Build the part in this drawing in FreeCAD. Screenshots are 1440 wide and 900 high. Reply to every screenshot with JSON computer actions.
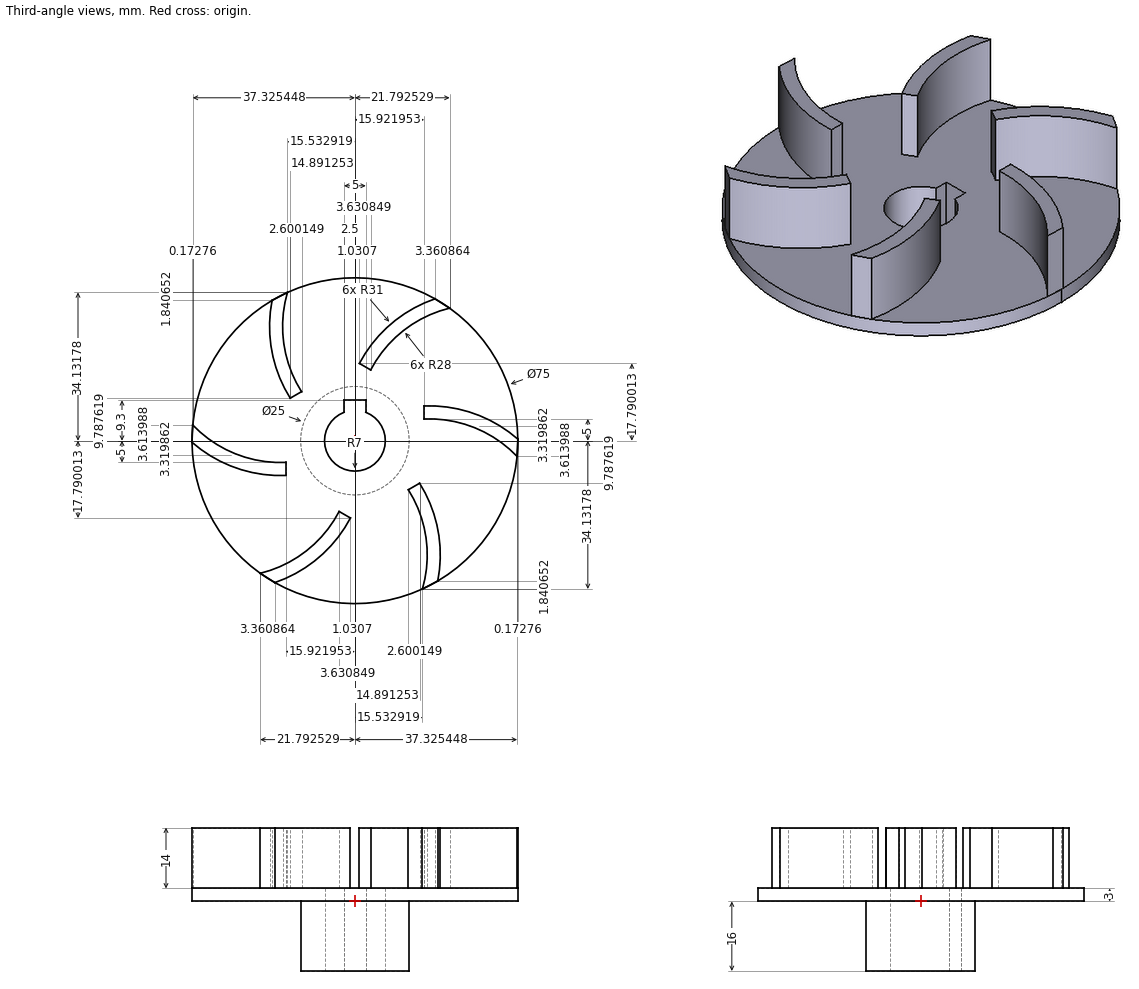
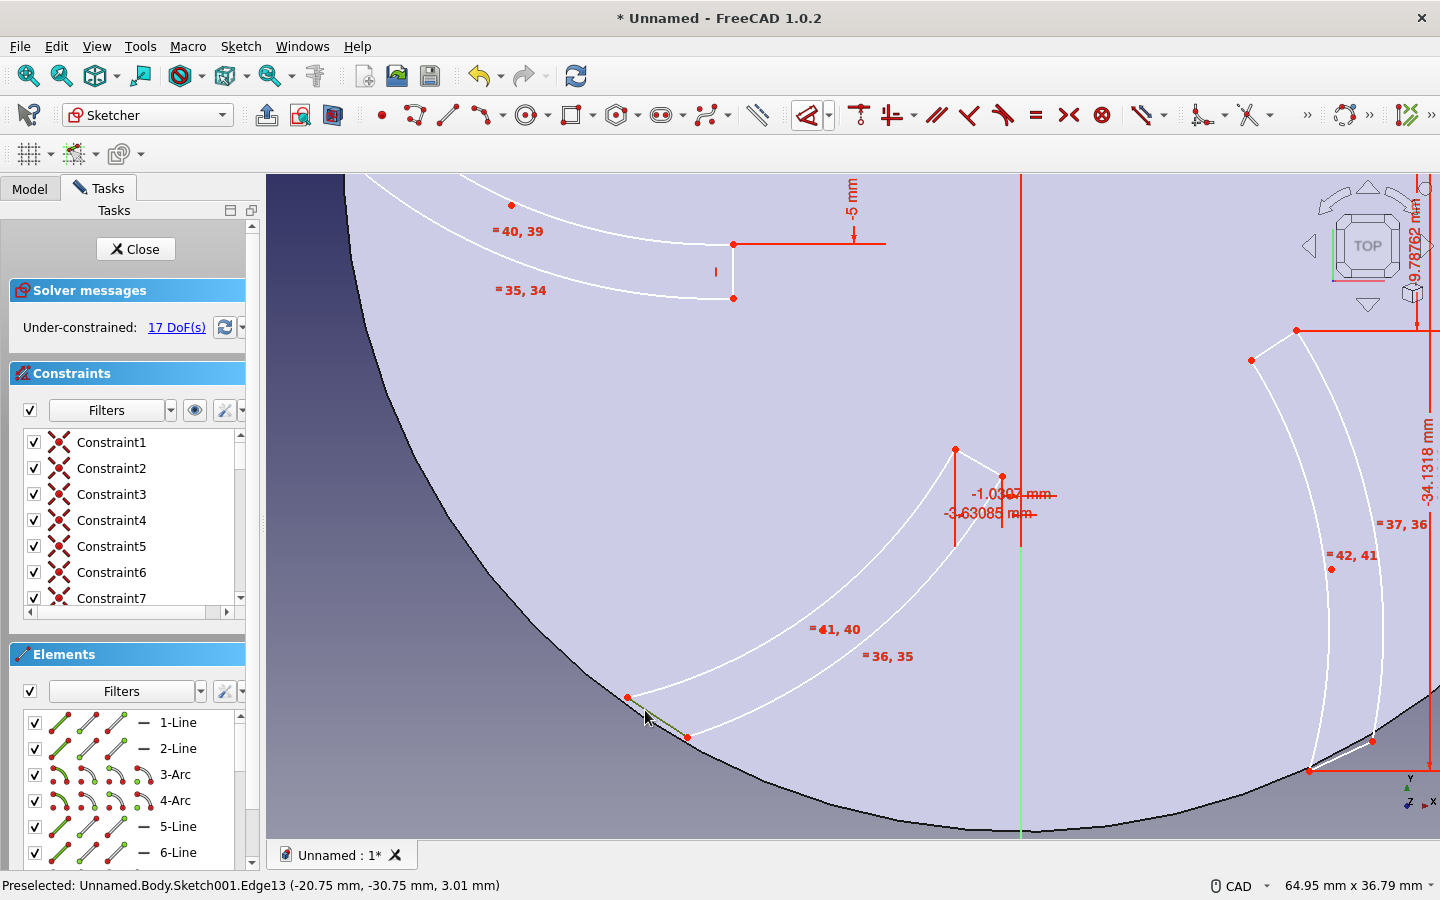
{"action": "key", "text": "l"}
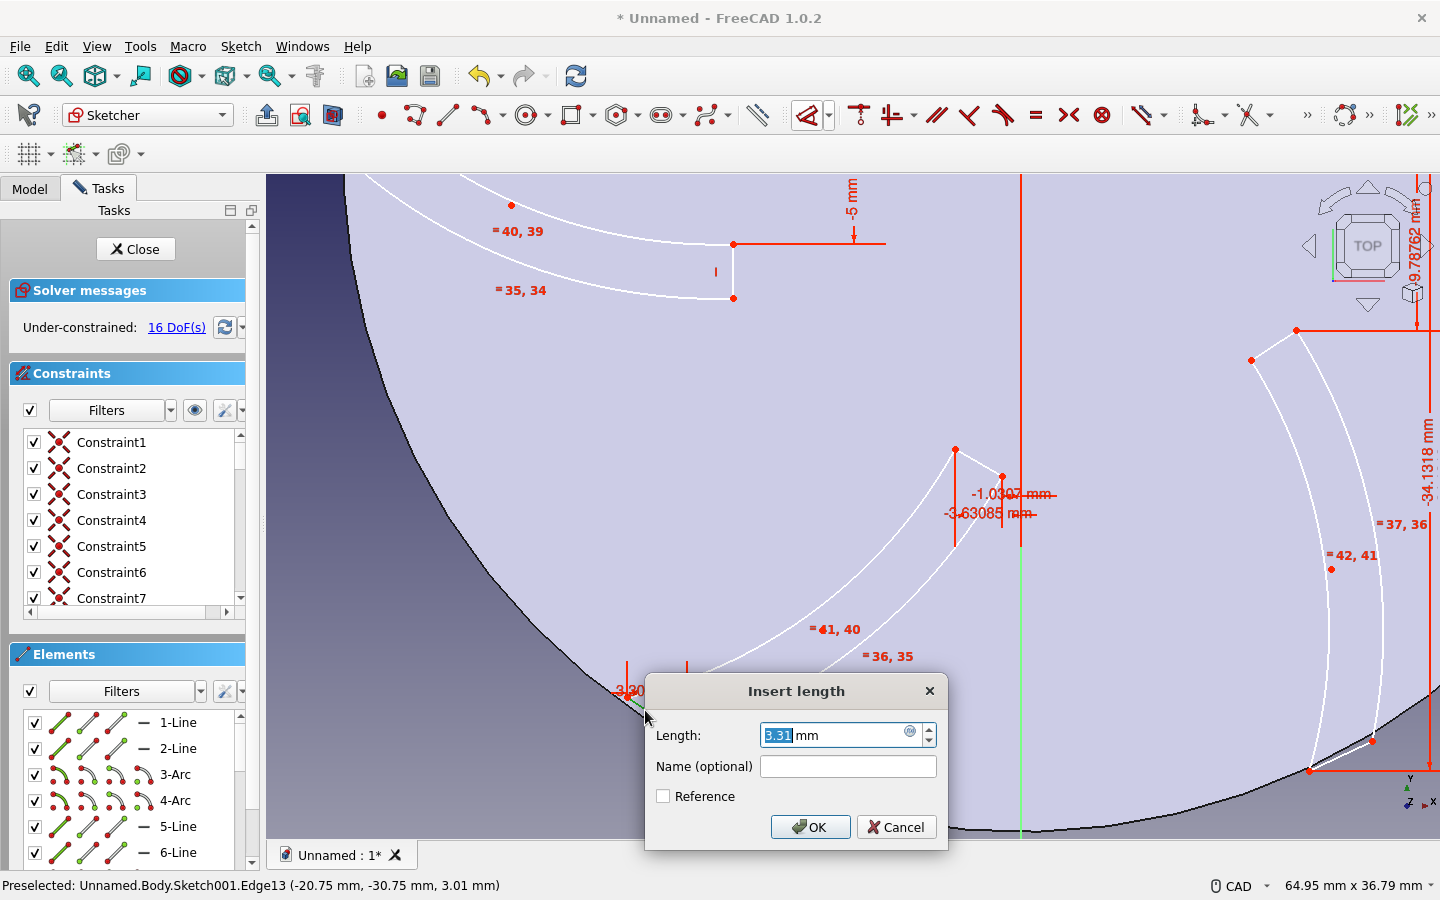
{"action": "type", "text": "3.360864"}
{"action": "key", "text": "Return"}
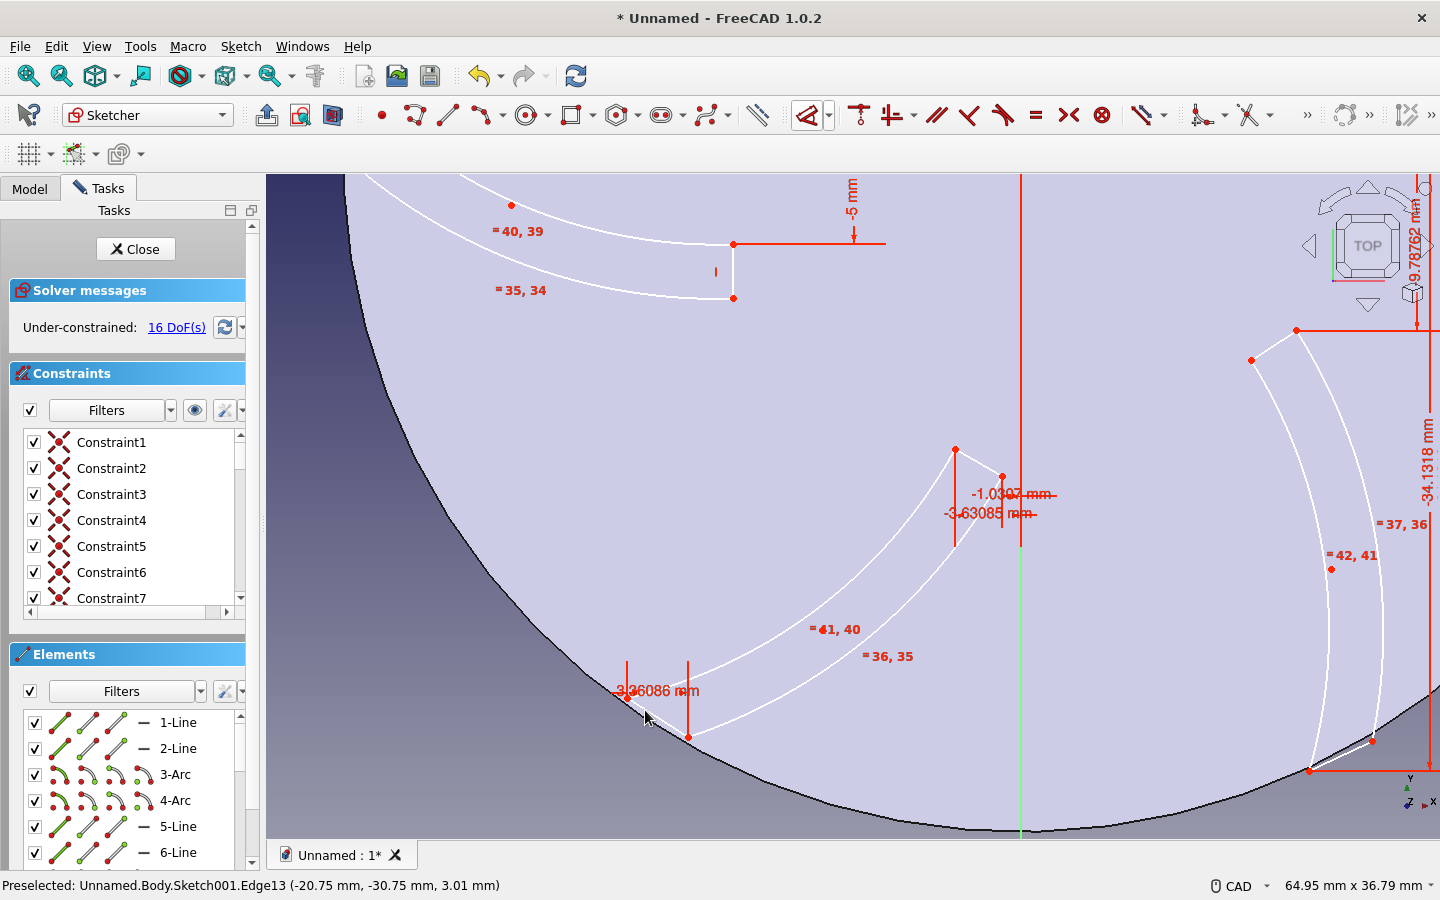
{"action": "scroll", "coordinate": [647, 712], "scroll_direction": "down", "scroll_amount": 5}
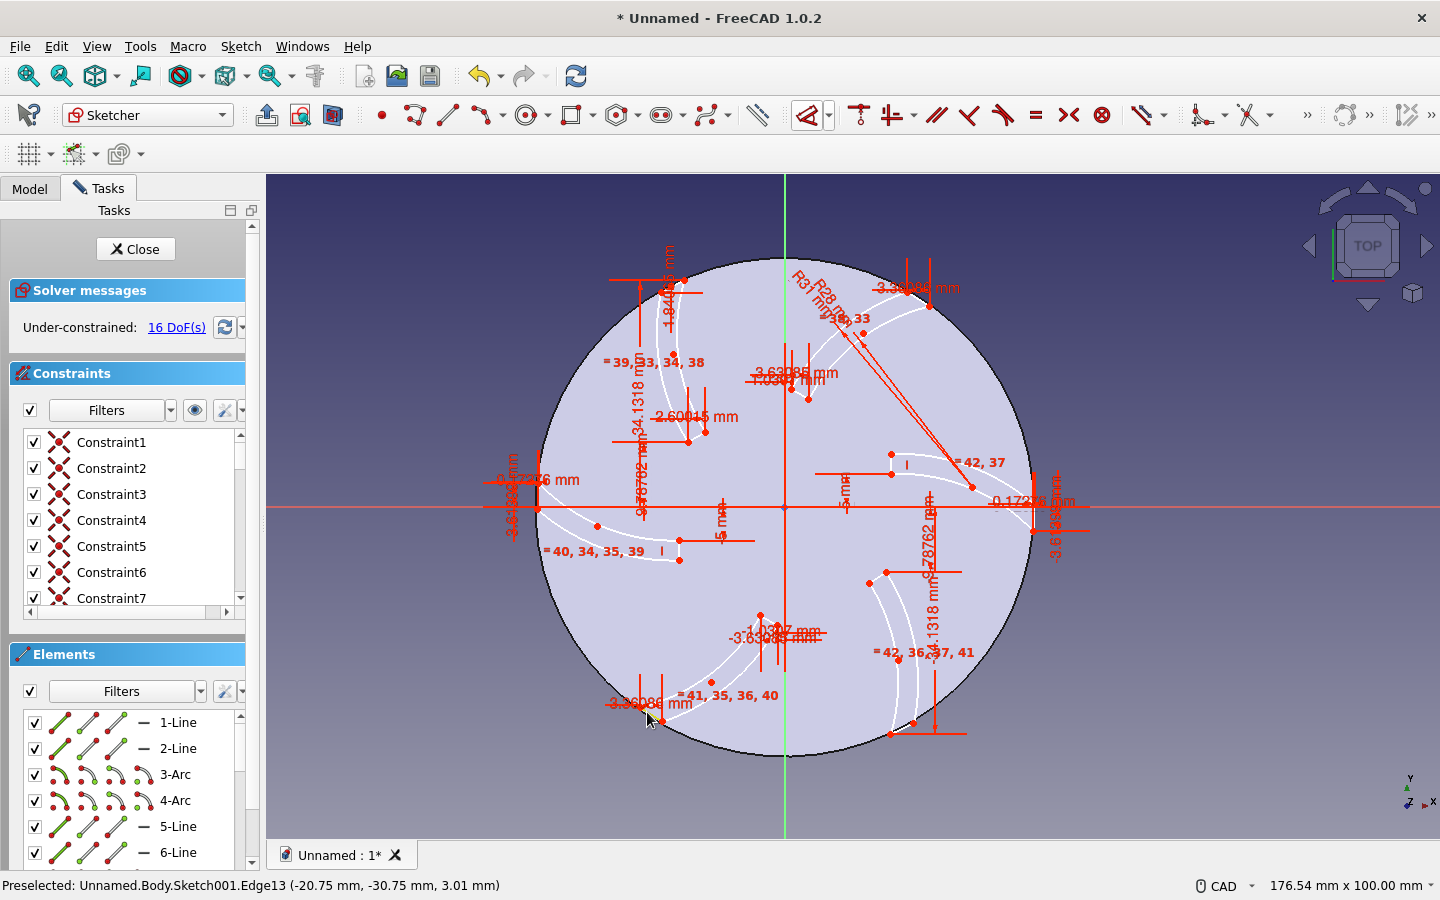
{"action": "scroll", "coordinate": [898, 731], "scroll_direction": "up", "scroll_amount": 6}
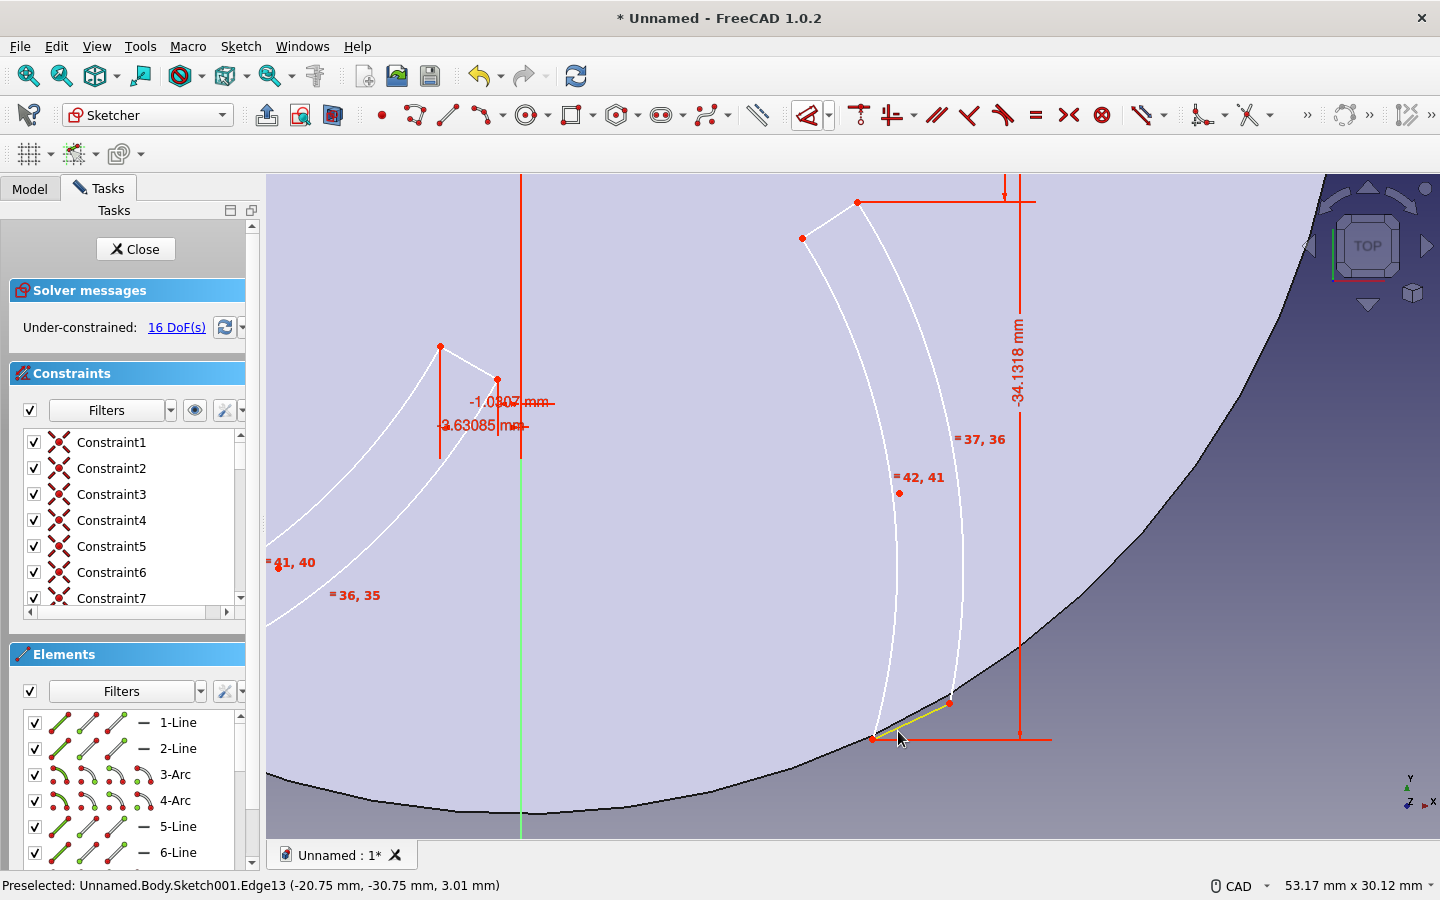
{"action": "left_click", "coordinate": [896, 729]}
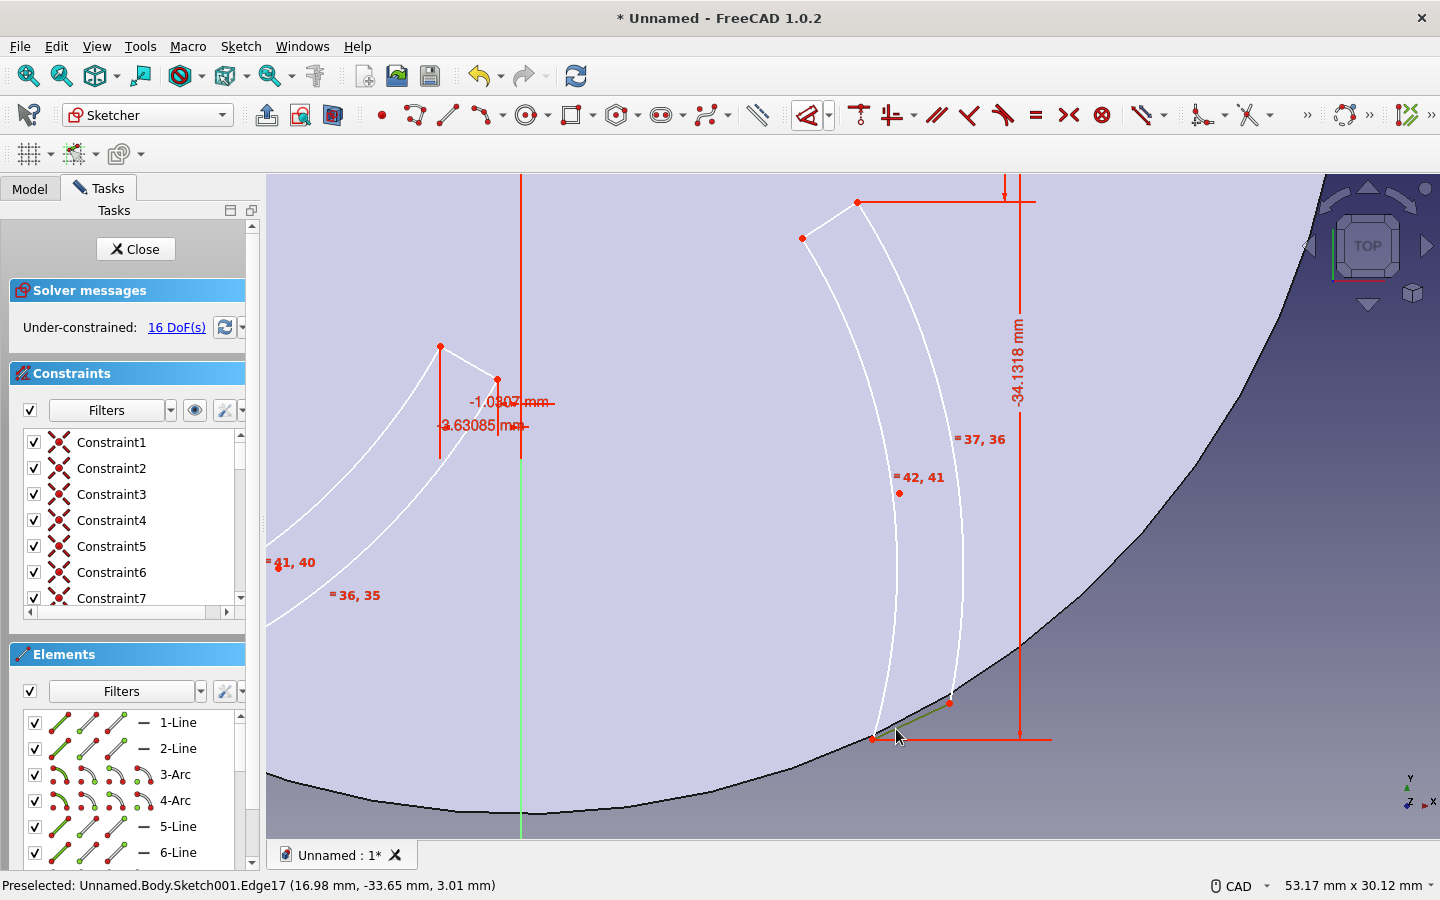
{"action": "key", "text": "i"}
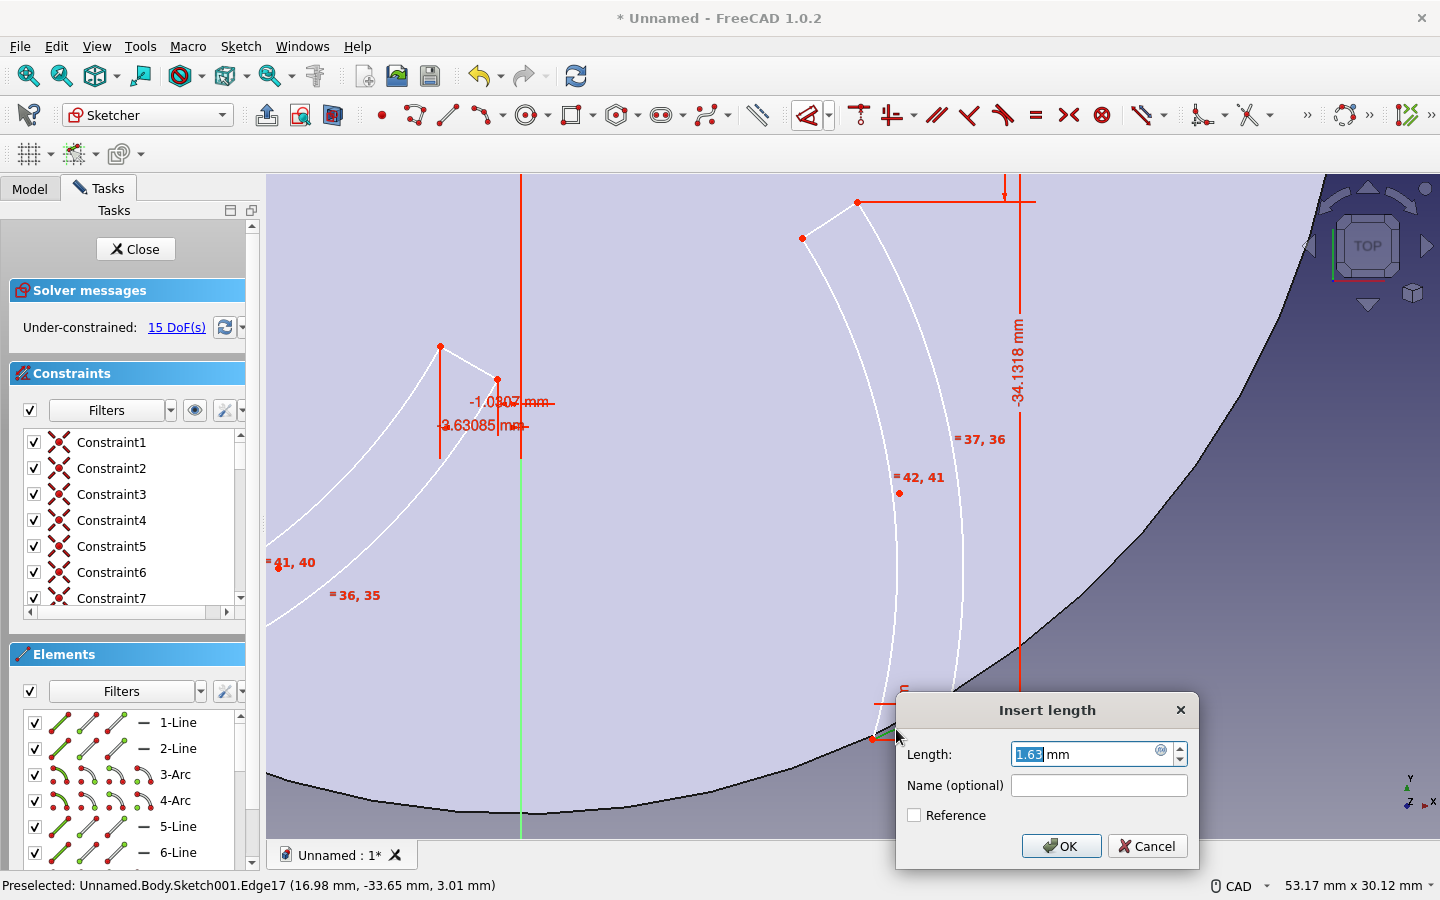
{"action": "type", "text": "1.840652"}
{"action": "key", "text": "Return"}